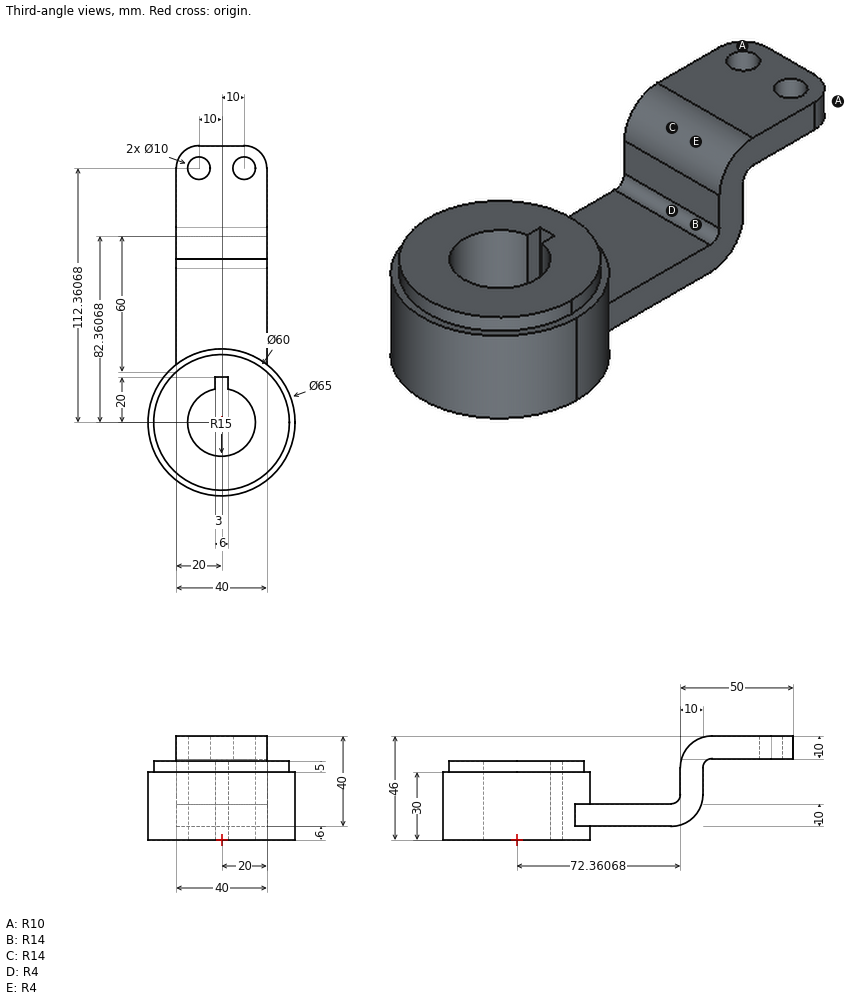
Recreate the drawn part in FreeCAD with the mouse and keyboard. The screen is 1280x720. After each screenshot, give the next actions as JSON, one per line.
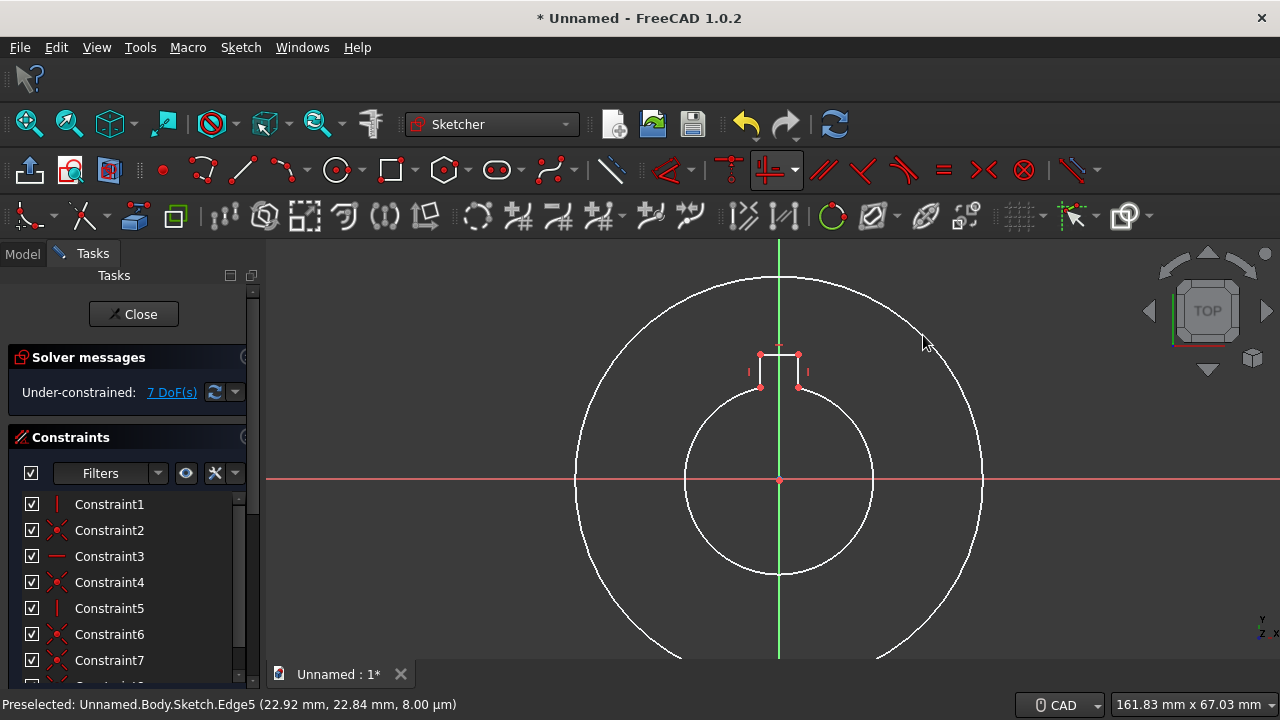
{"action": "left_click_drag", "start_coordinate": [769, 469], "coordinate": [789, 490]}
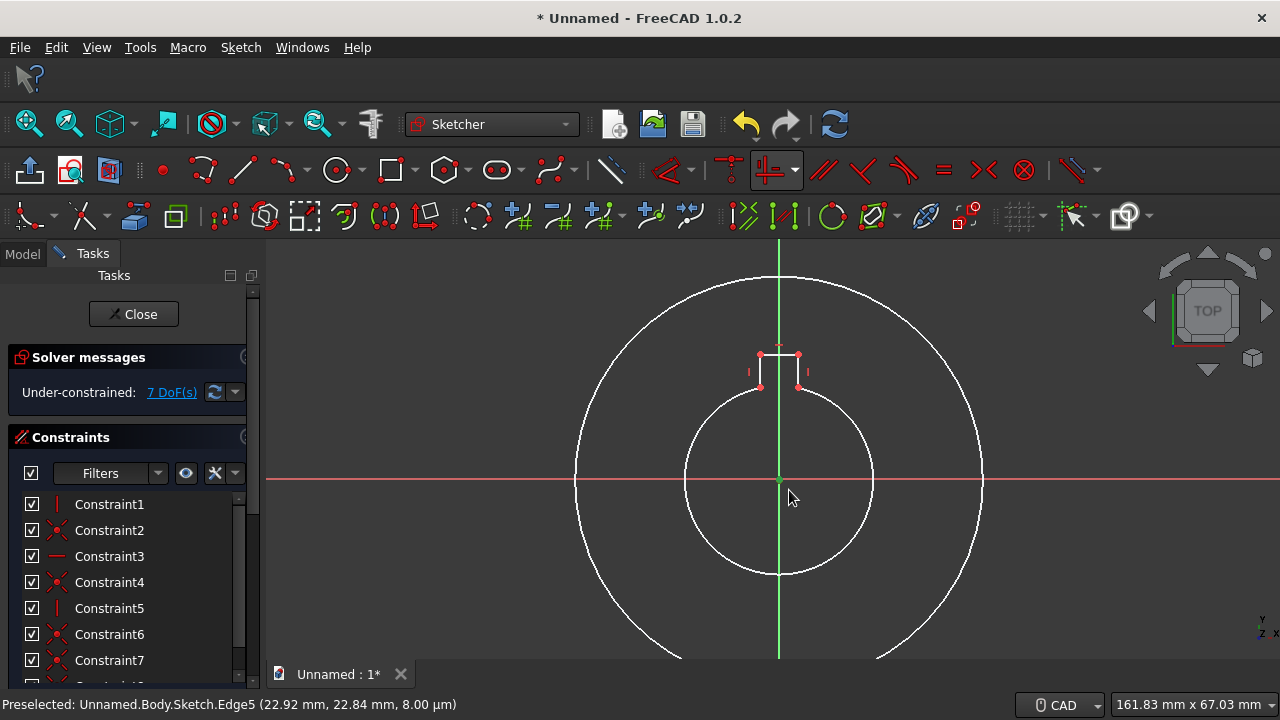
{"action": "key", "text": "c"}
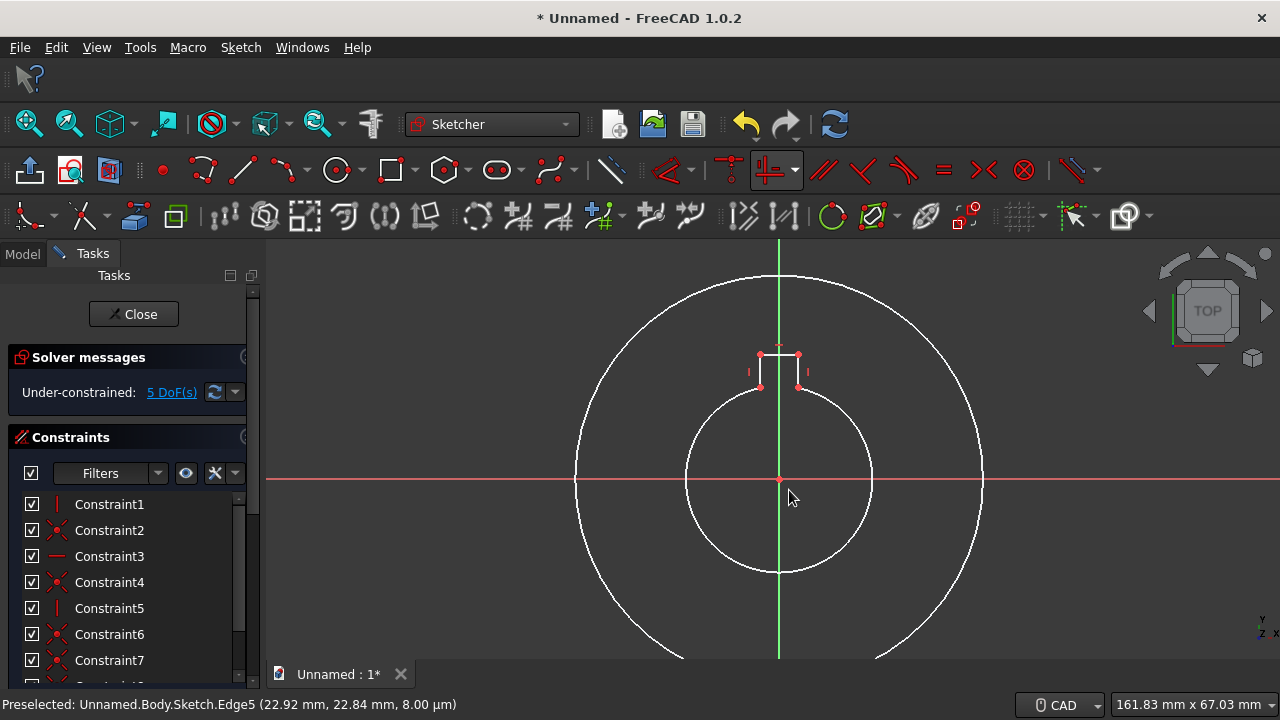
{"action": "key", "text": "d"}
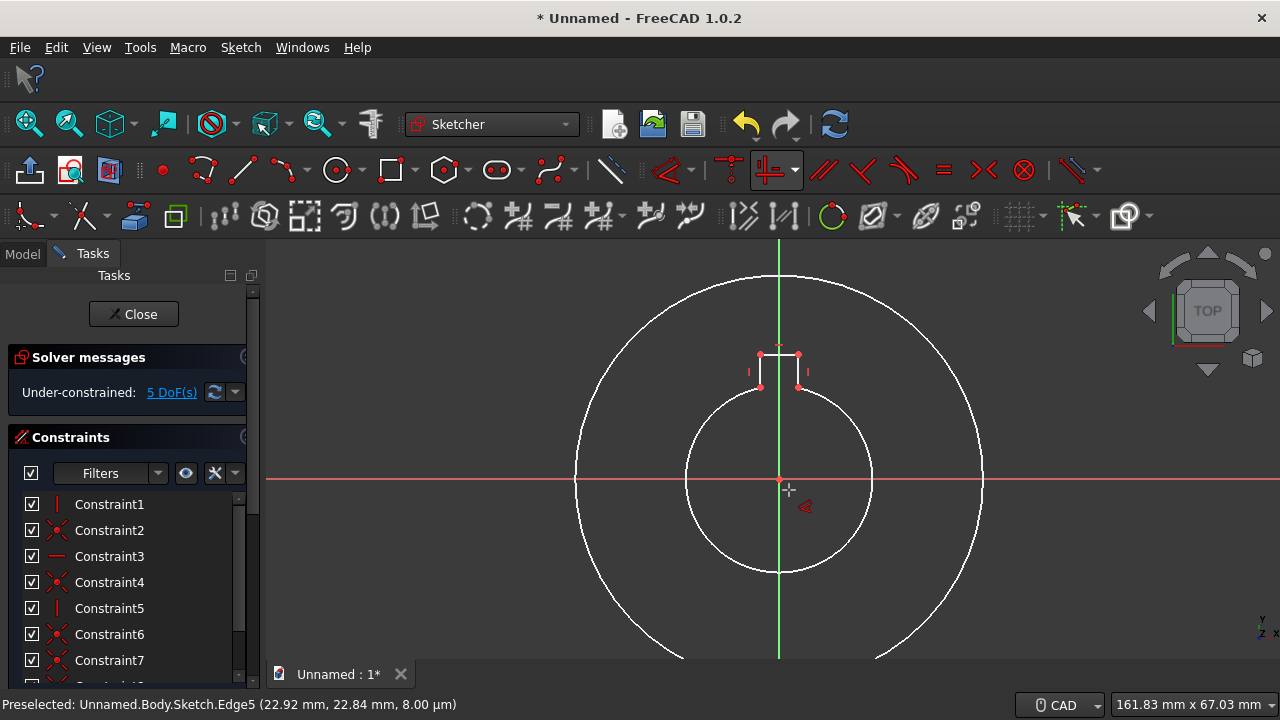
{"action": "left_click", "coordinate": [693, 515]}
{"action": "left_click", "coordinate": [663, 527]}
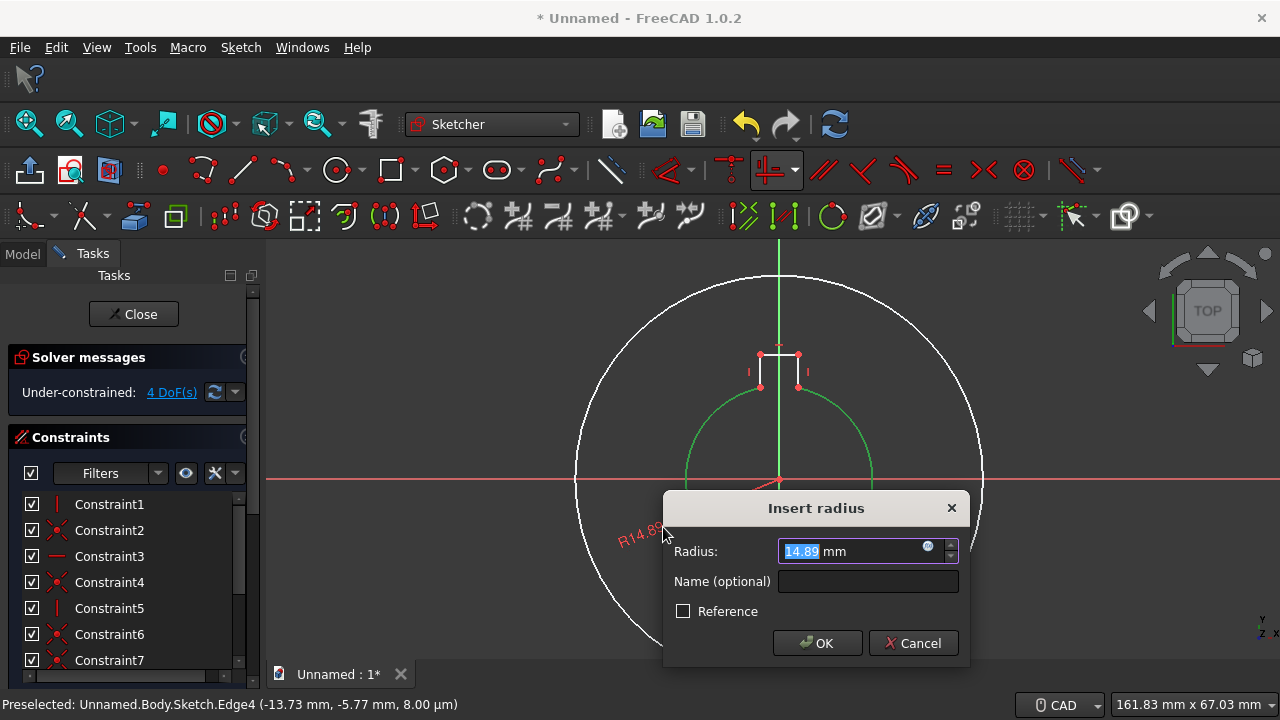
{"action": "type", "text": "15"}
{"action": "key", "text": "Return"}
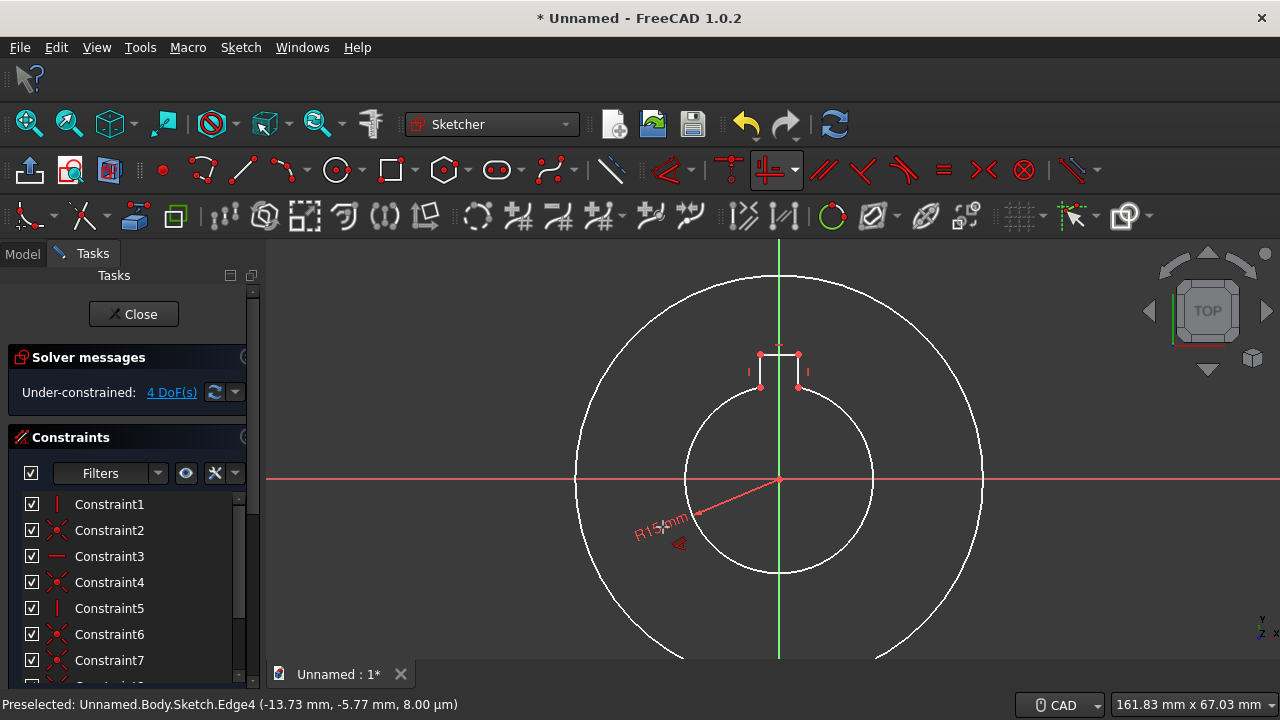
{"action": "left_click", "coordinate": [923, 335]}
{"action": "left_click", "coordinate": [946, 312]}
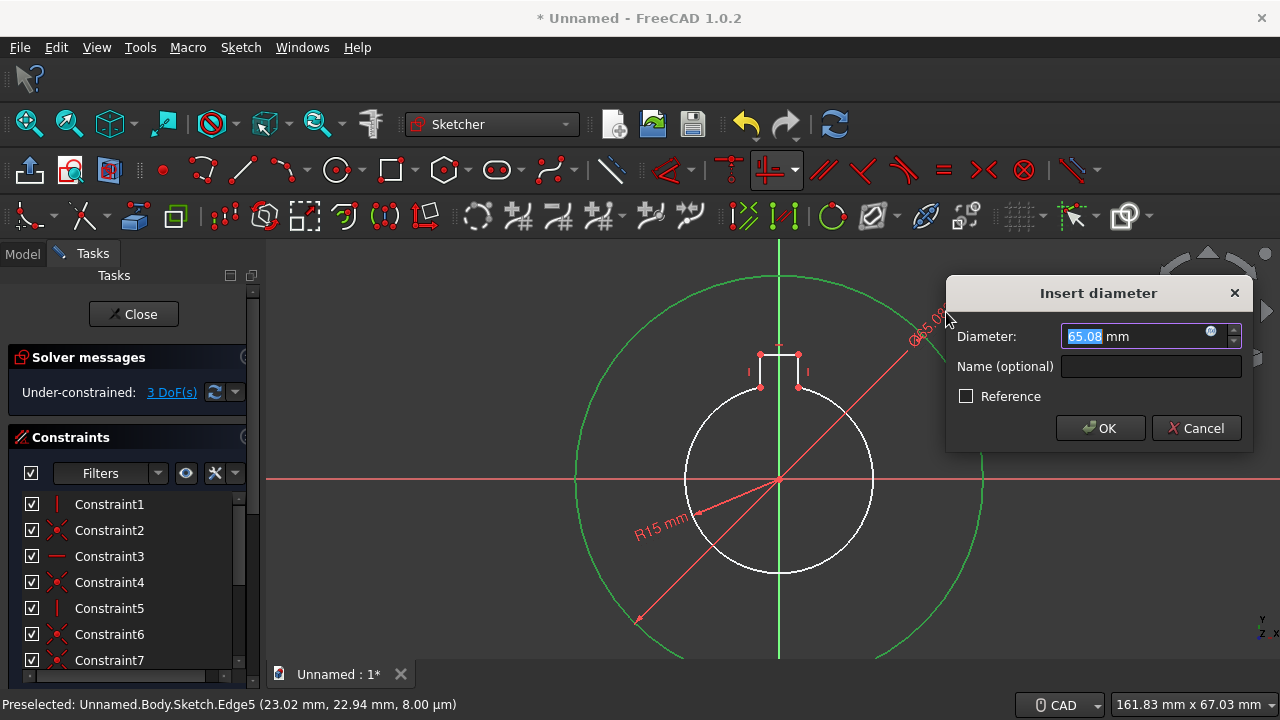
{"action": "type", "text": "65"}
{"action": "key", "text": "Return"}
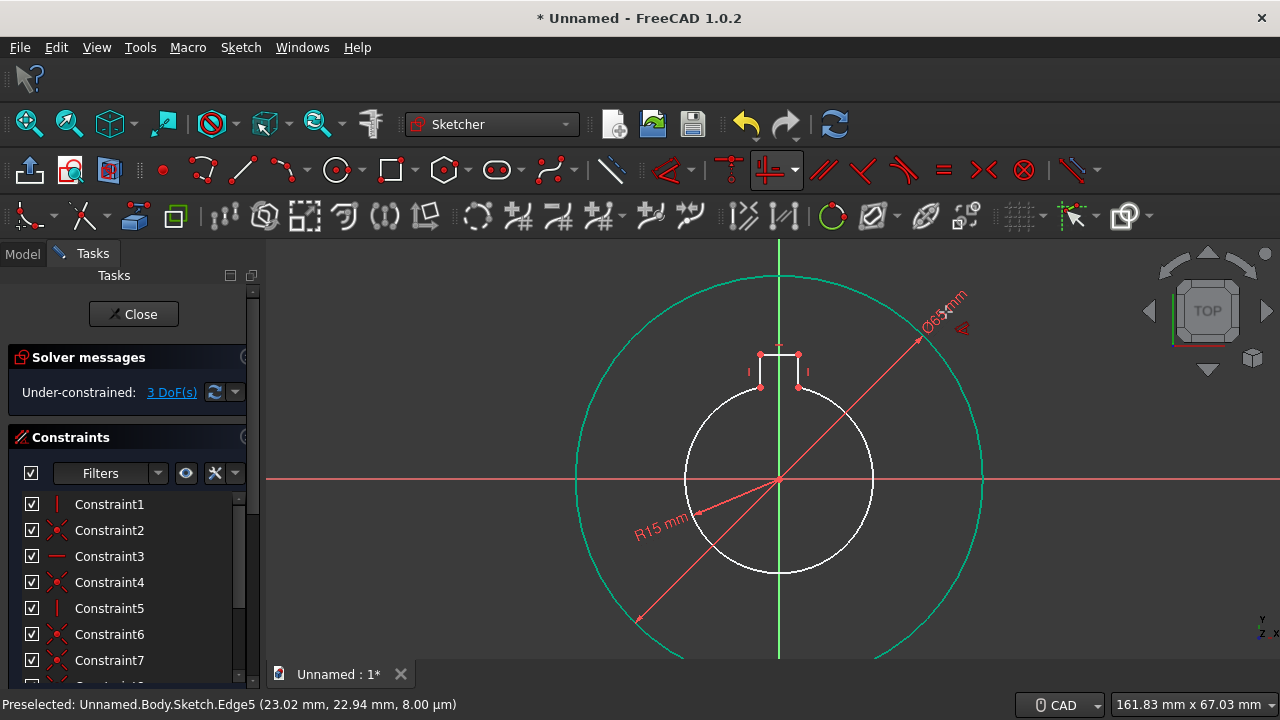
{"action": "left_click", "coordinate": [775, 355]}
{"action": "left_click", "coordinate": [766, 321]}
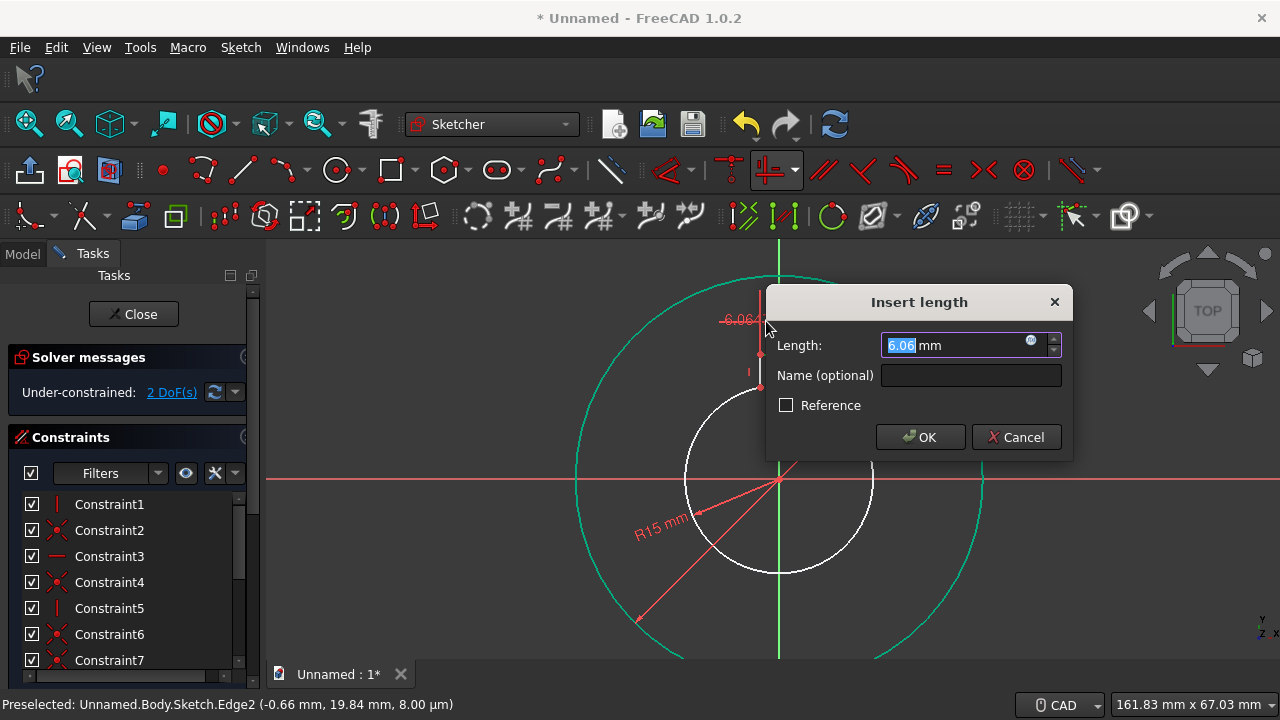
{"action": "type", "text": "6"}
{"action": "key", "text": "Return"}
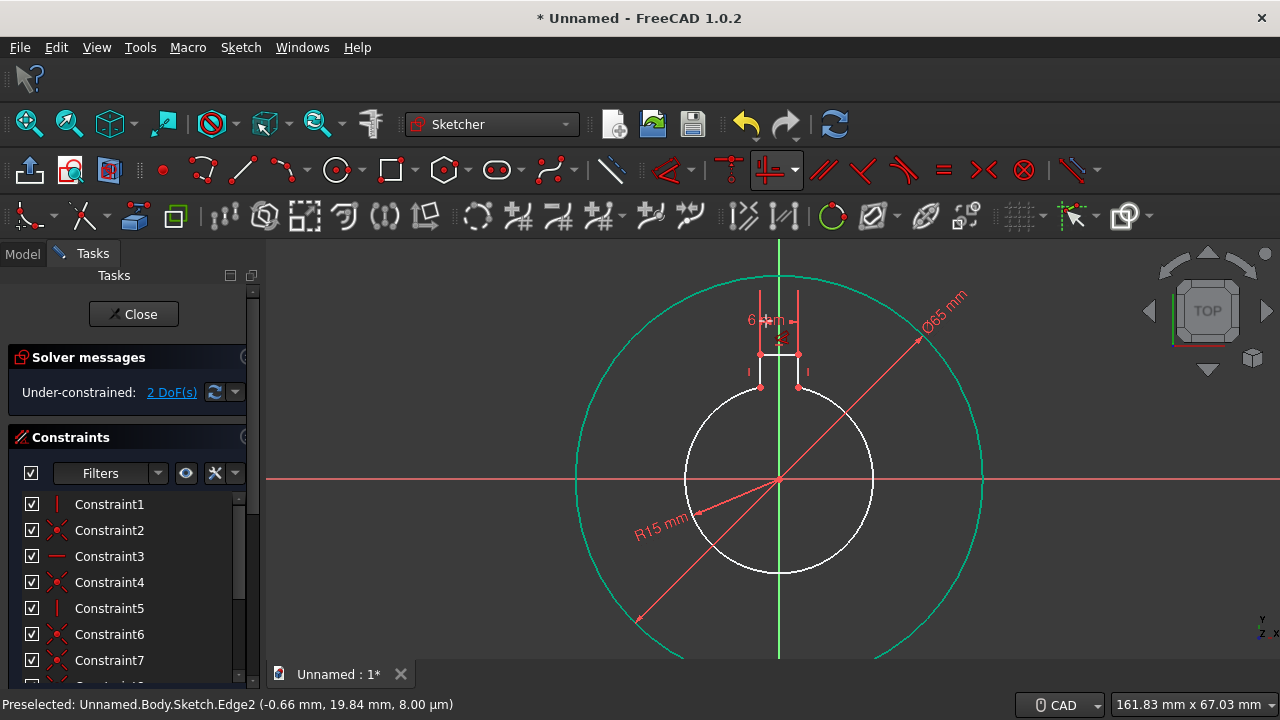
{"action": "scroll", "coordinate": [760, 387], "scroll_direction": "up", "scroll_amount": 4}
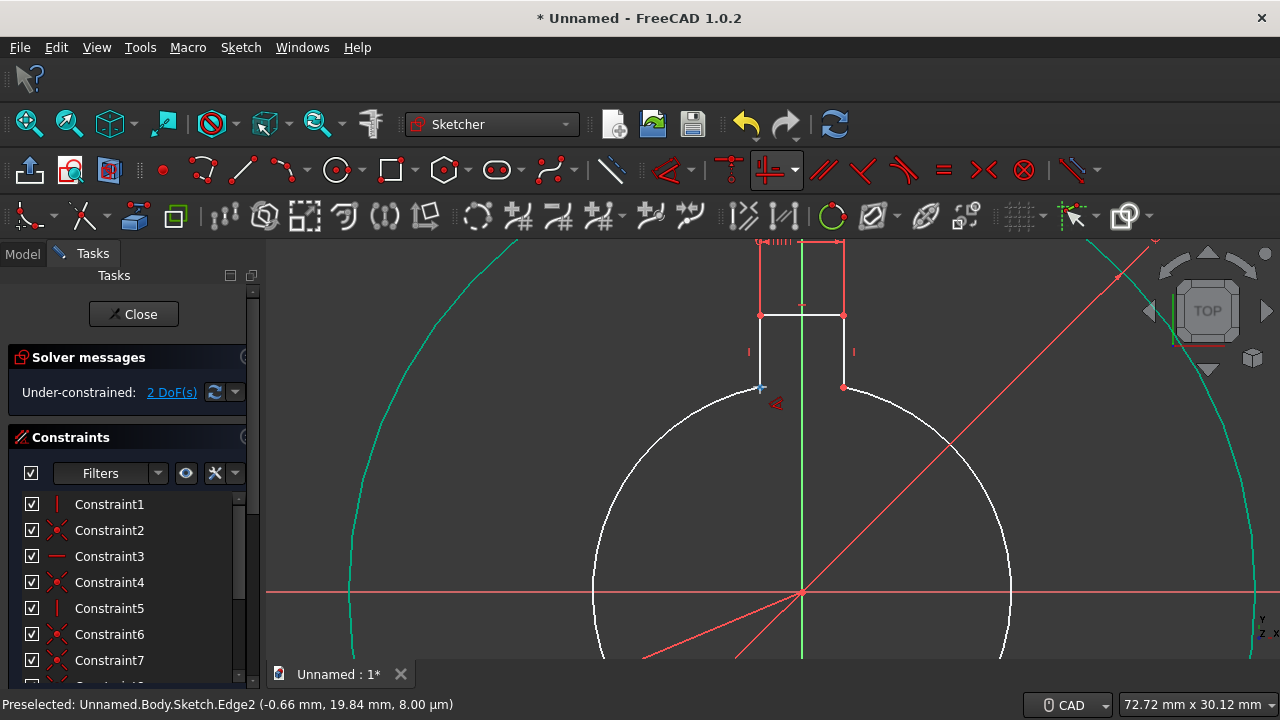
{"action": "left_click", "coordinate": [760, 387]}
{"action": "left_click", "coordinate": [781, 353]}